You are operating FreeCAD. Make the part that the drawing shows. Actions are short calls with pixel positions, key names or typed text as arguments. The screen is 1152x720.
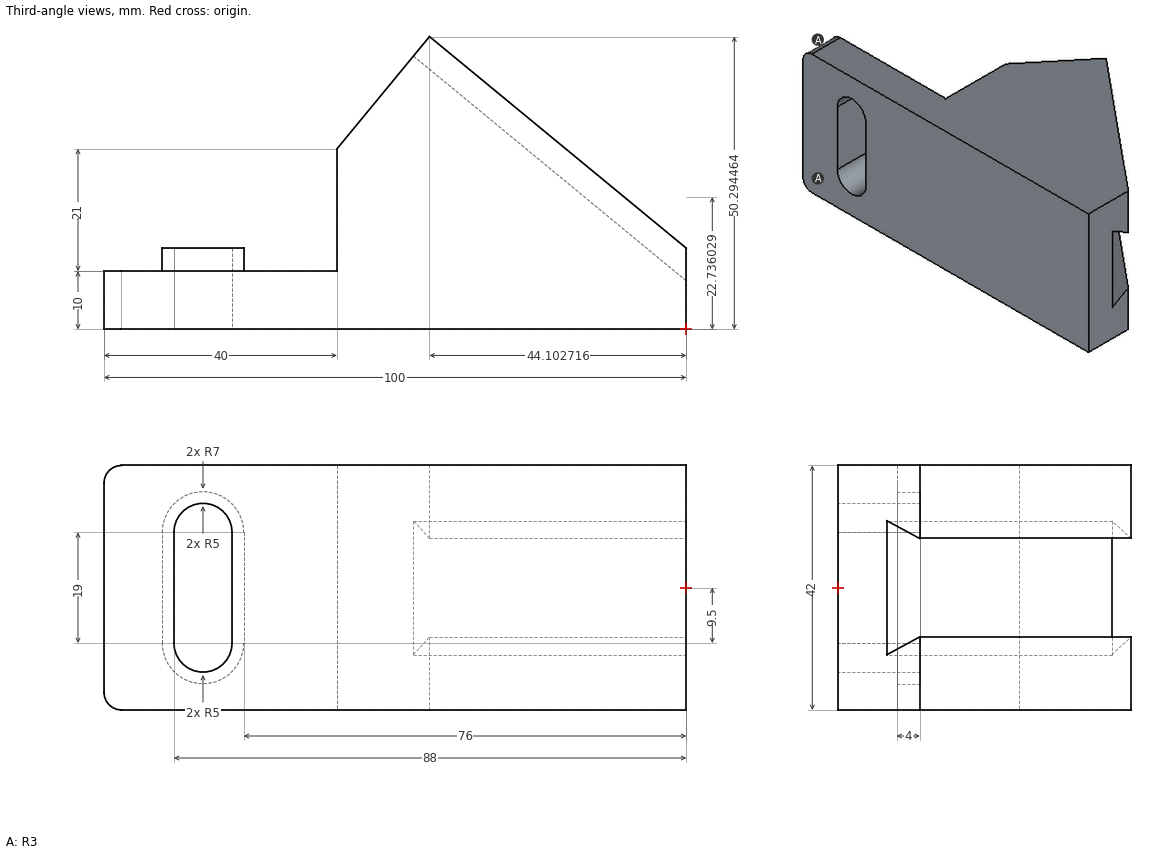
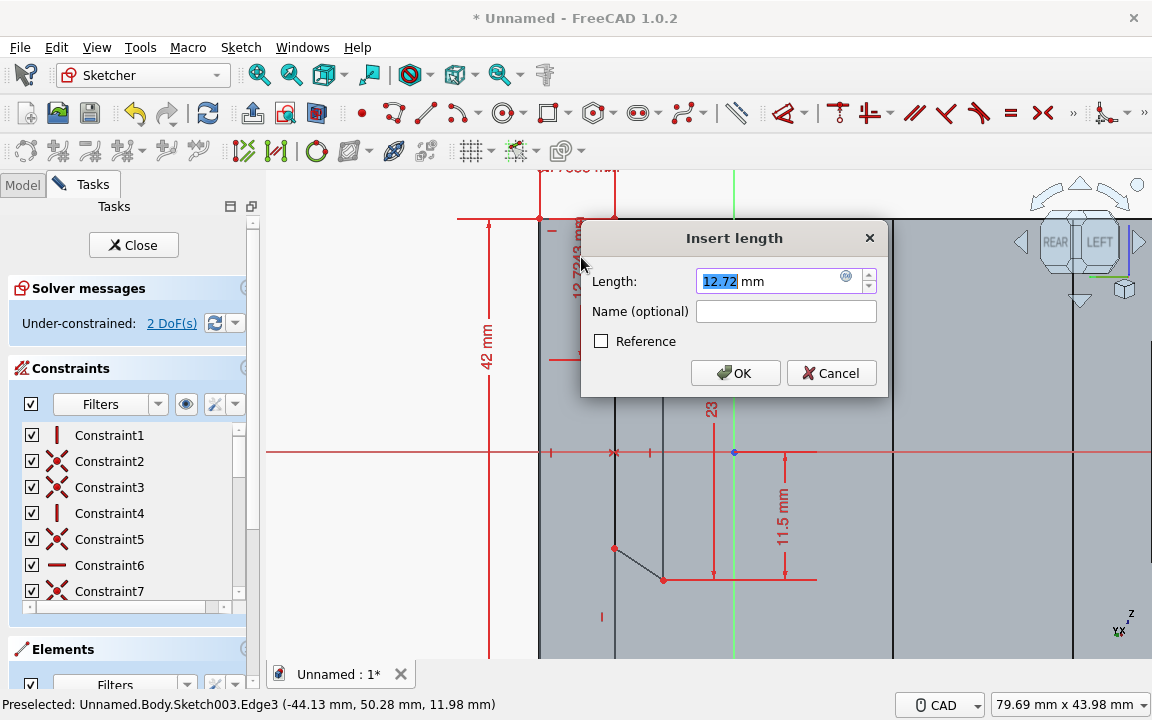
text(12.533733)
key(Return)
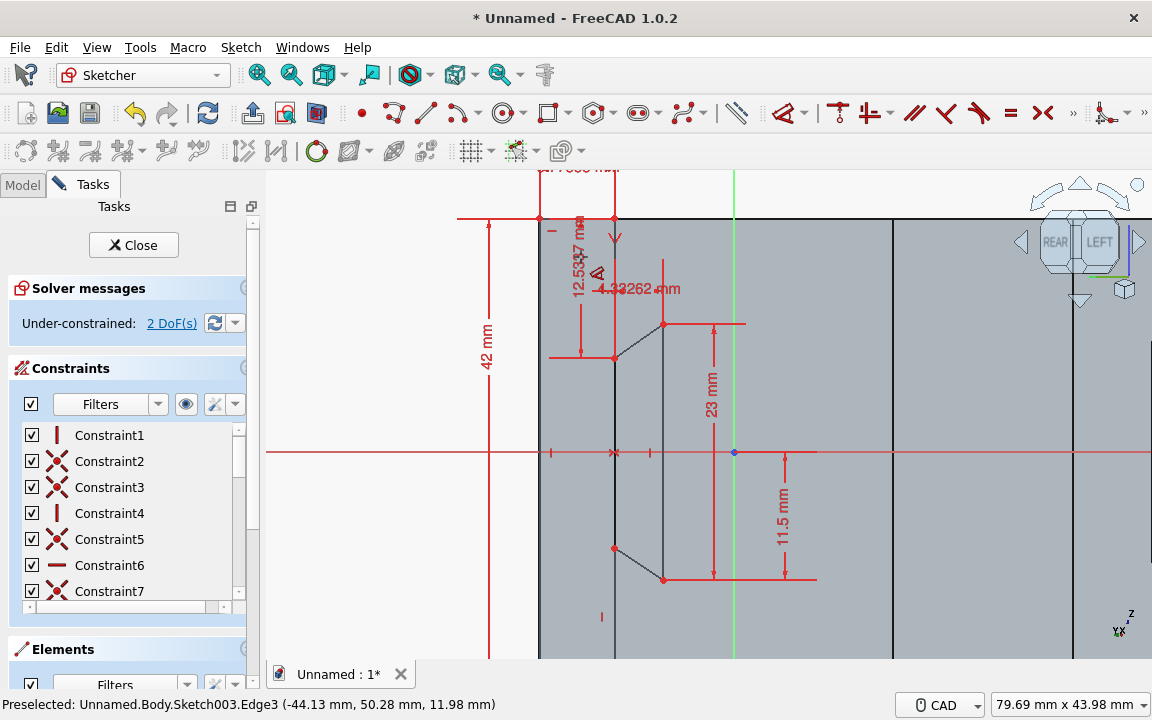
click(615, 589)
click(581, 590)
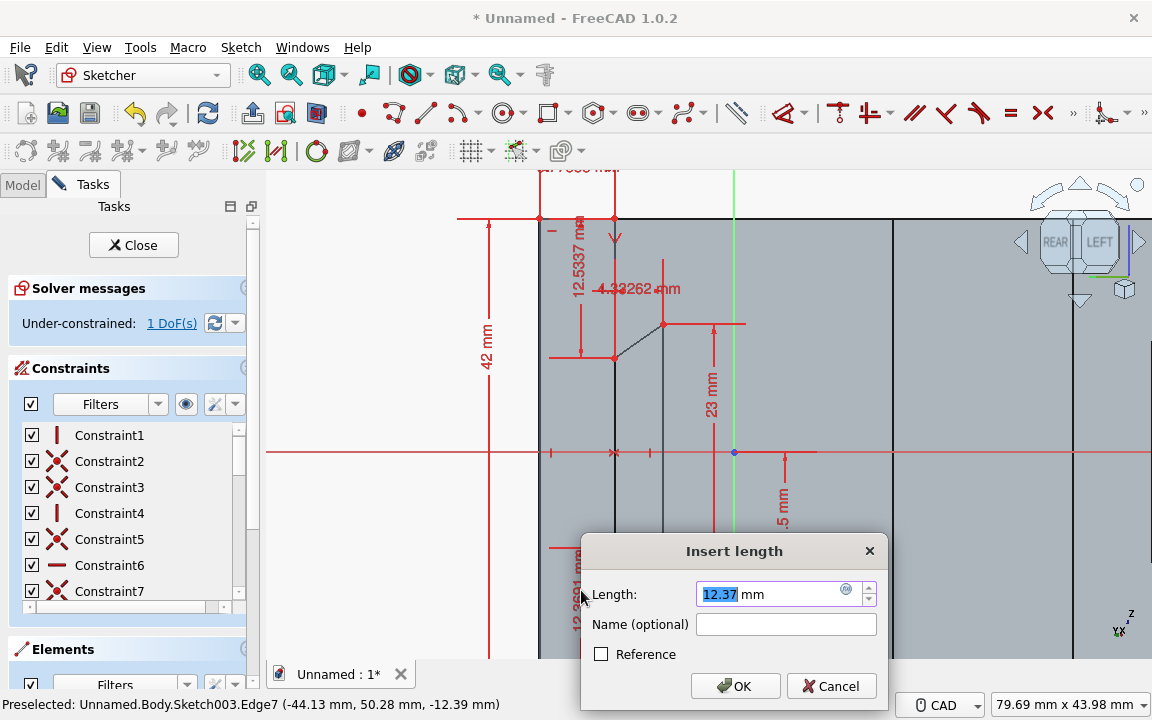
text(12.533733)
key(Return)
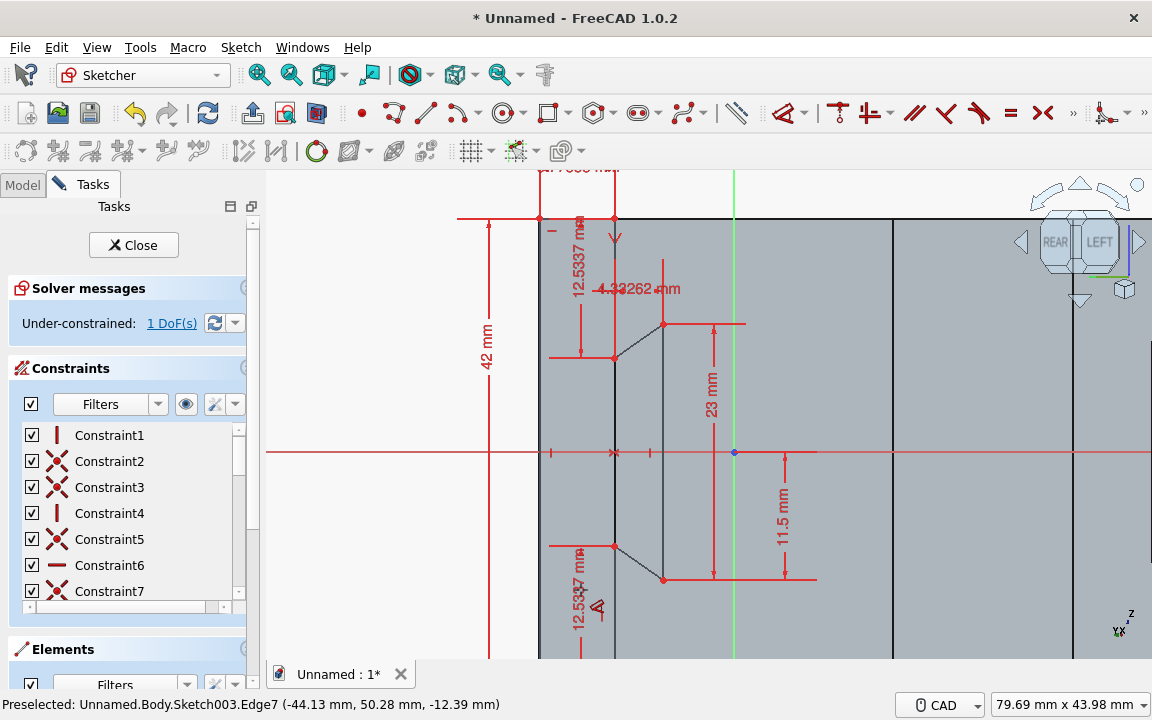
click(663, 580)
click(699, 614)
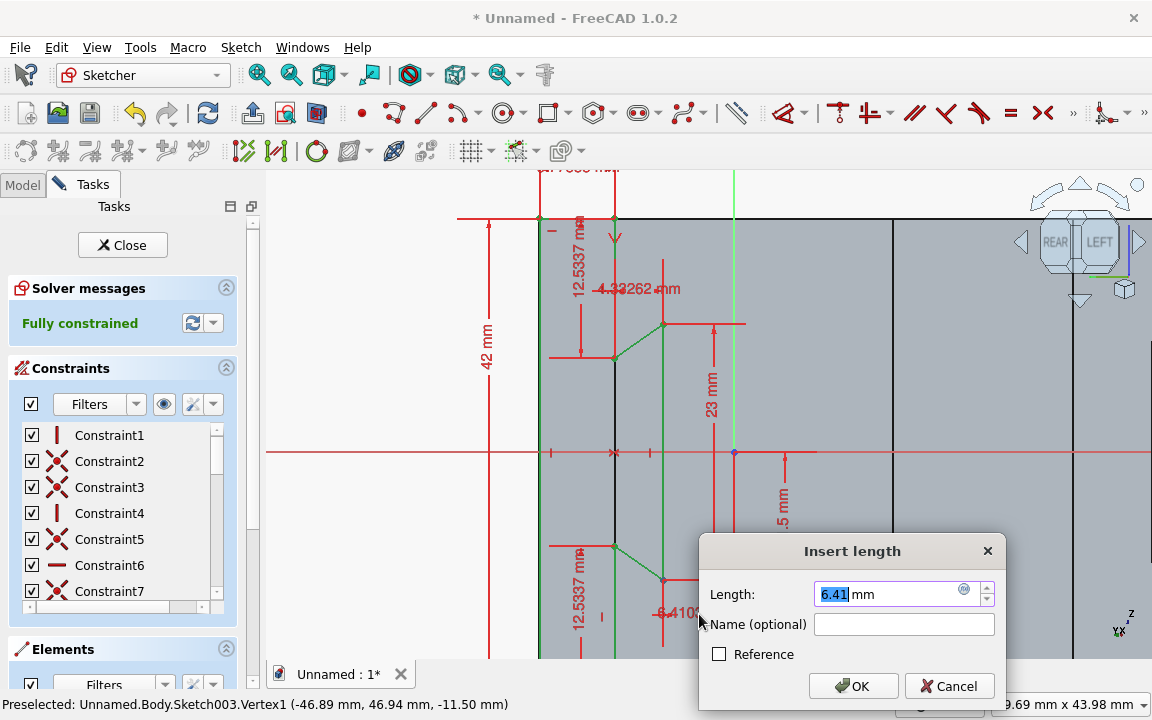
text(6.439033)
key(Return)
key(Escape)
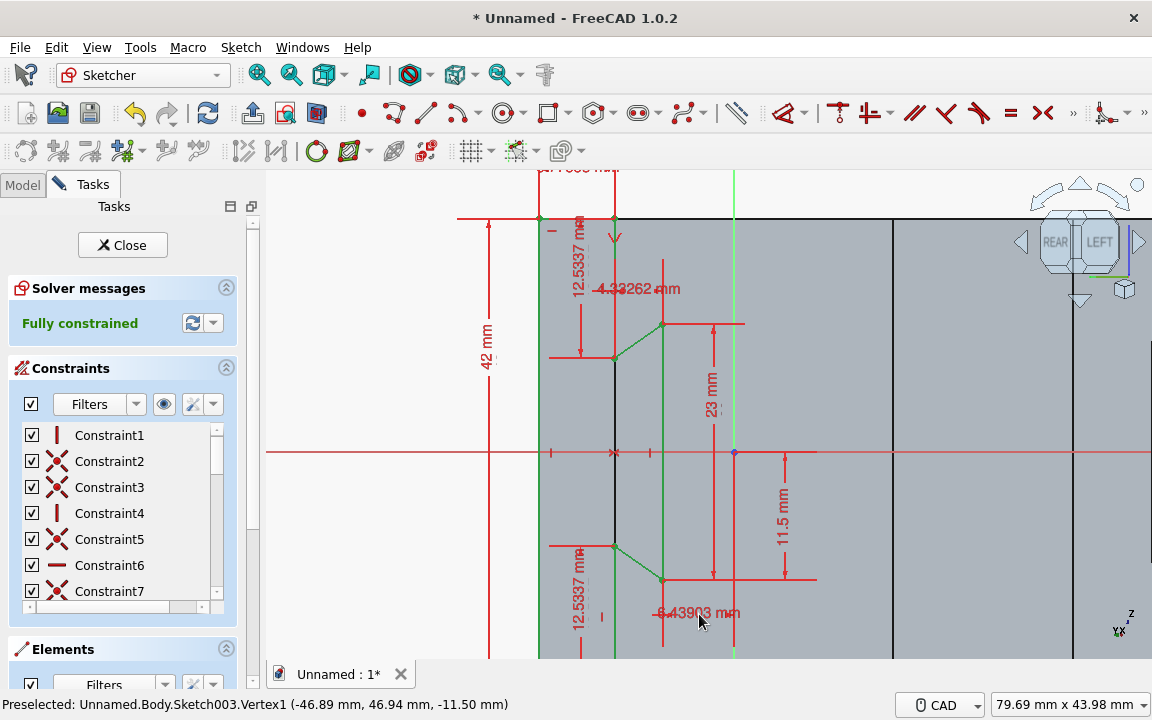
click(123, 245)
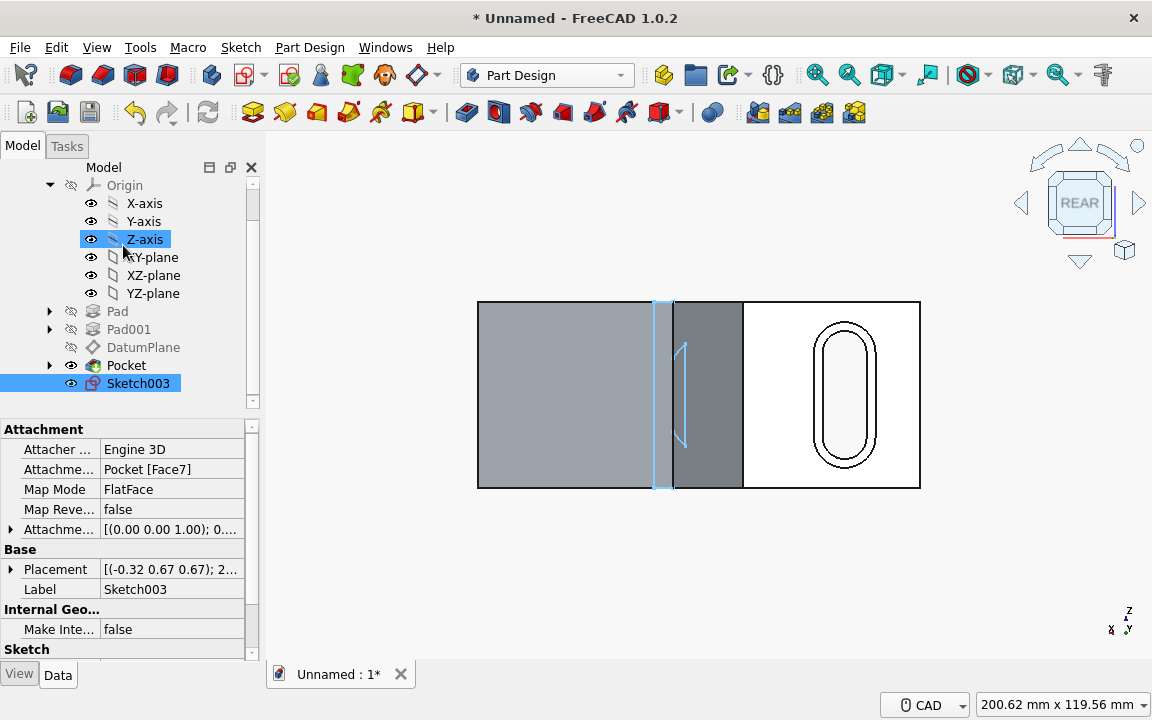
click(468, 112)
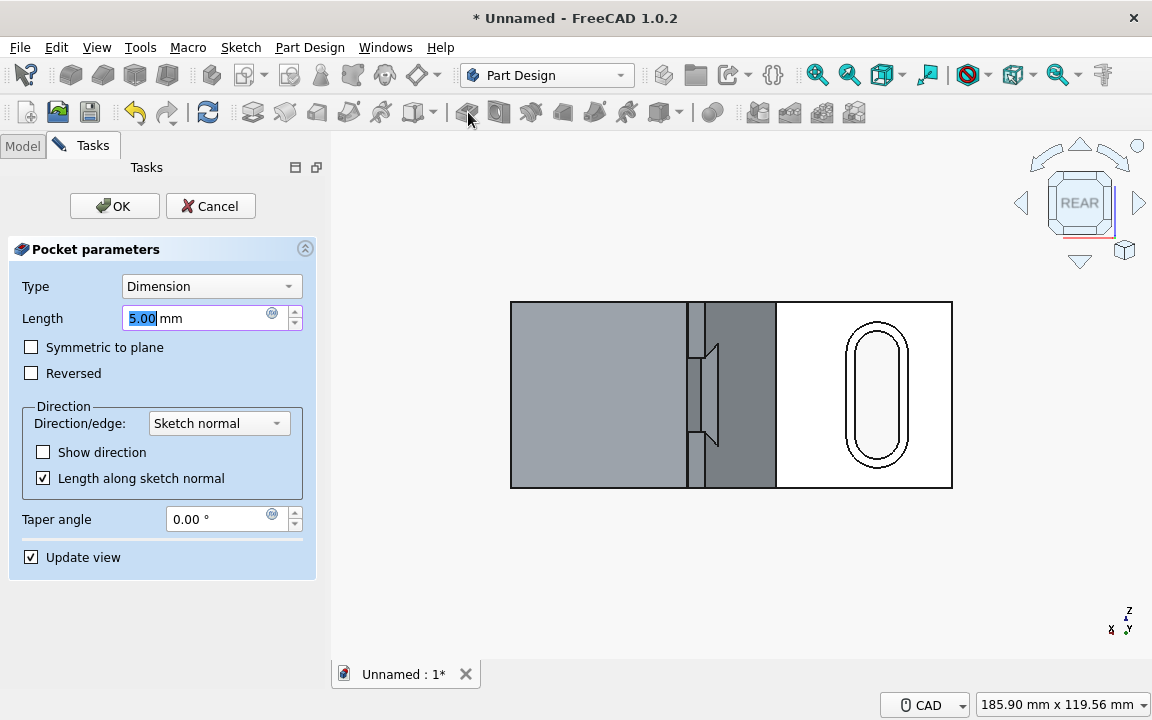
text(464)
key(Tab)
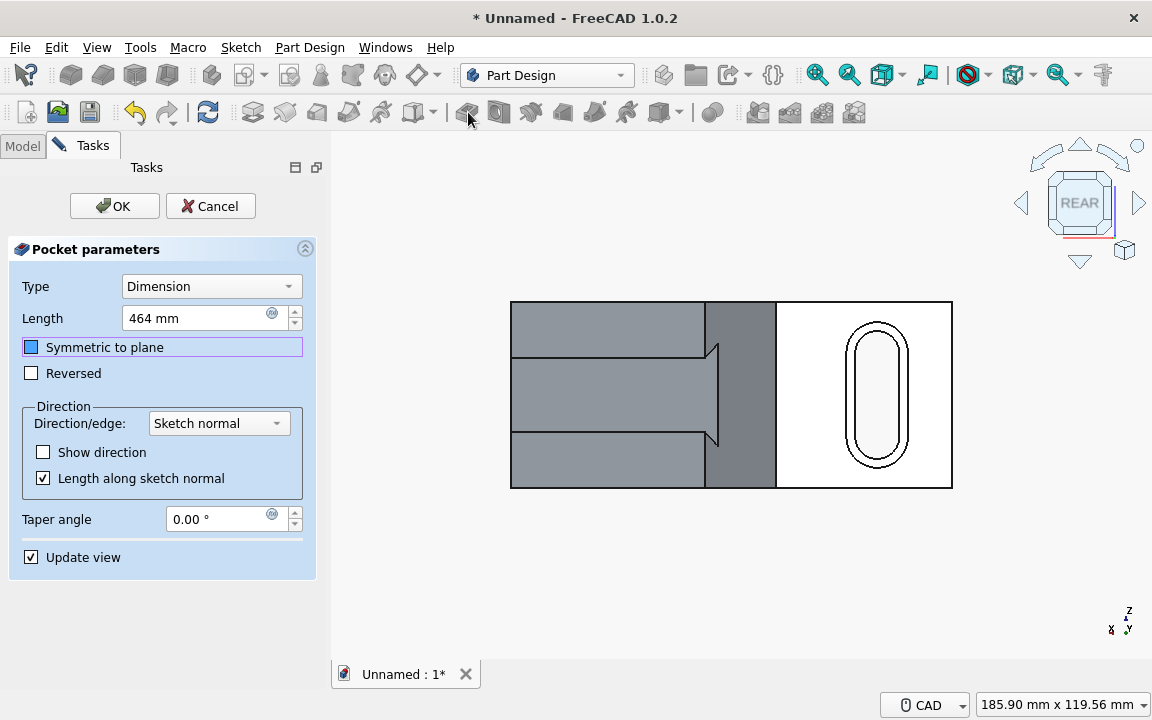
click(115, 206)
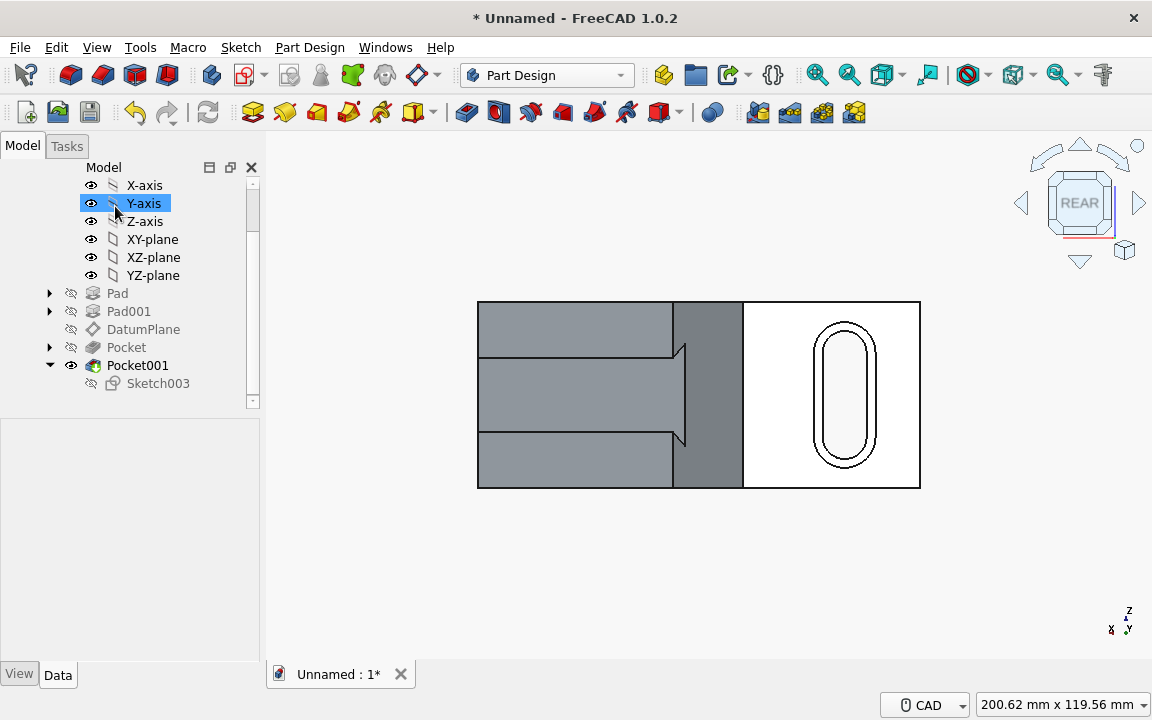
key(0)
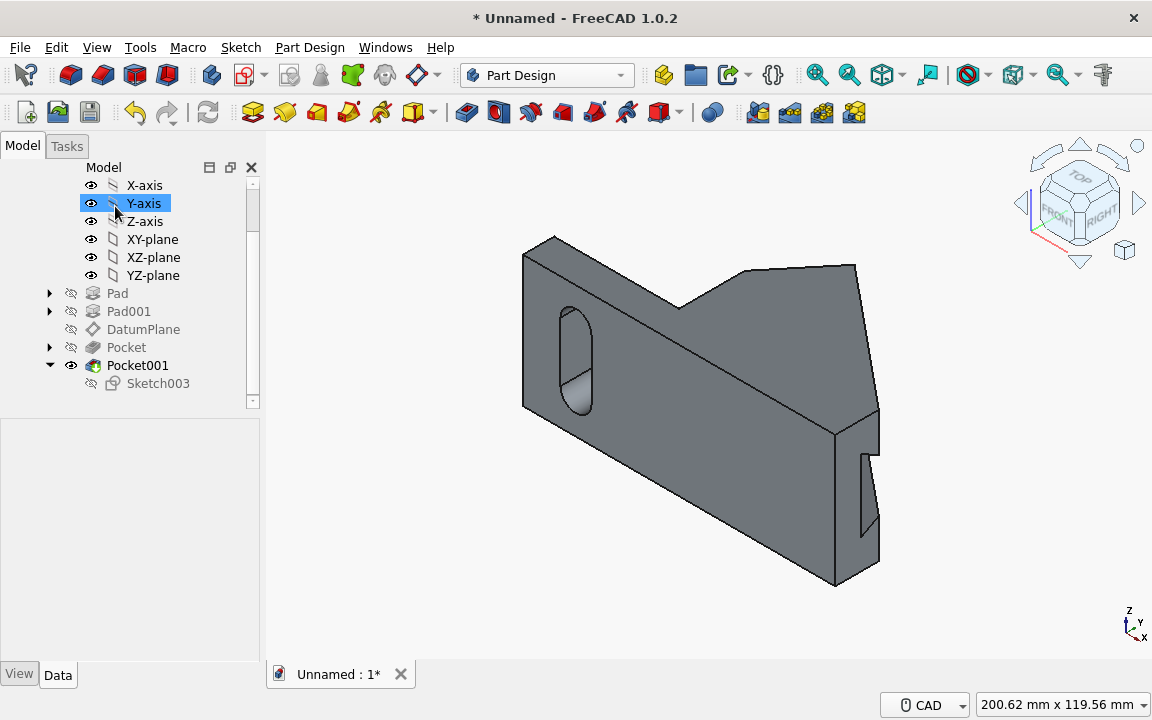
key(2)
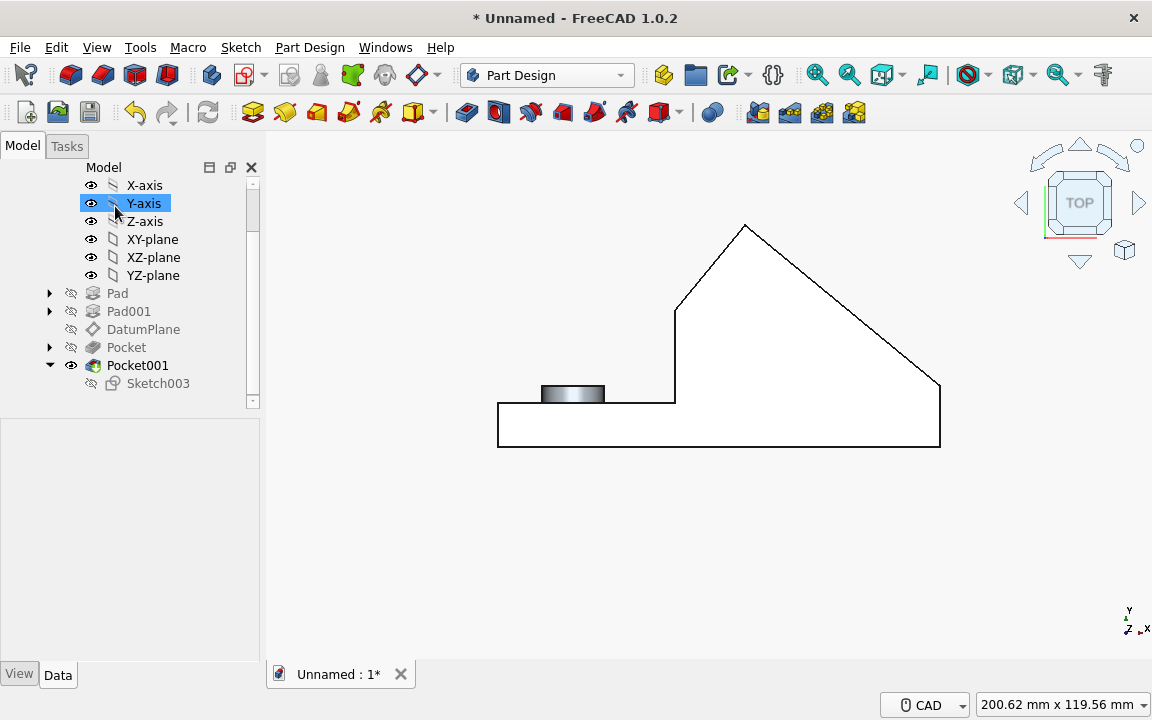
click(498, 424)